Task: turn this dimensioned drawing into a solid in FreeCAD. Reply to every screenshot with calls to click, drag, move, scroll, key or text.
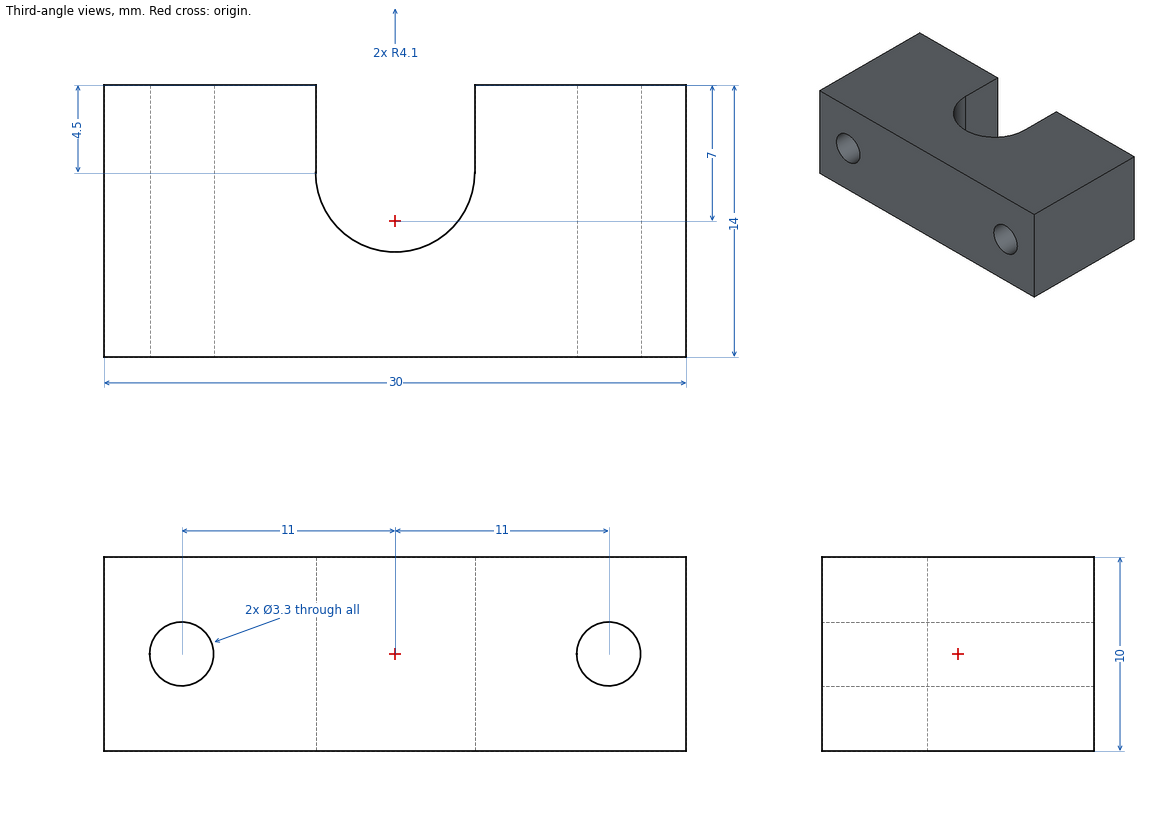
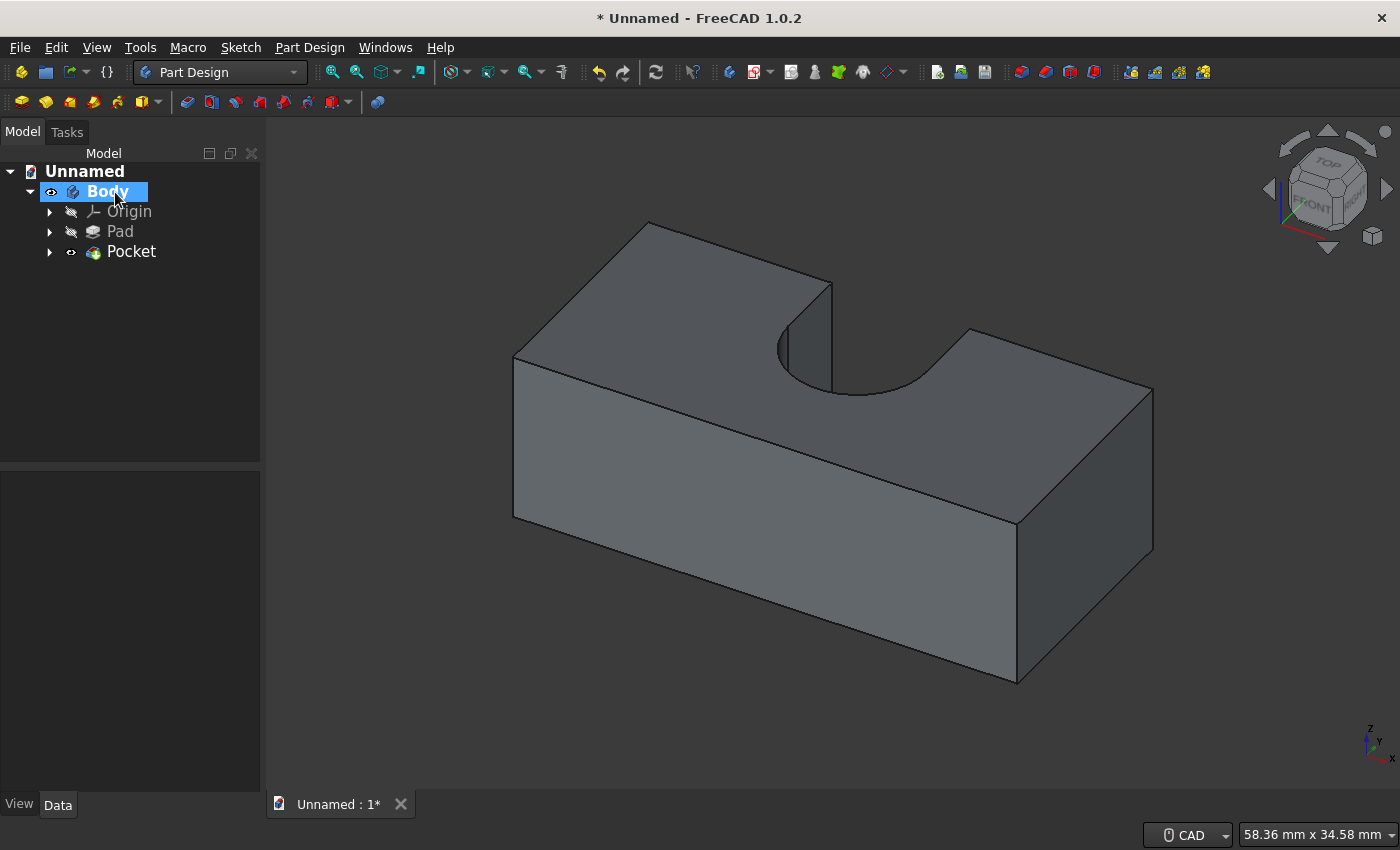
key(4)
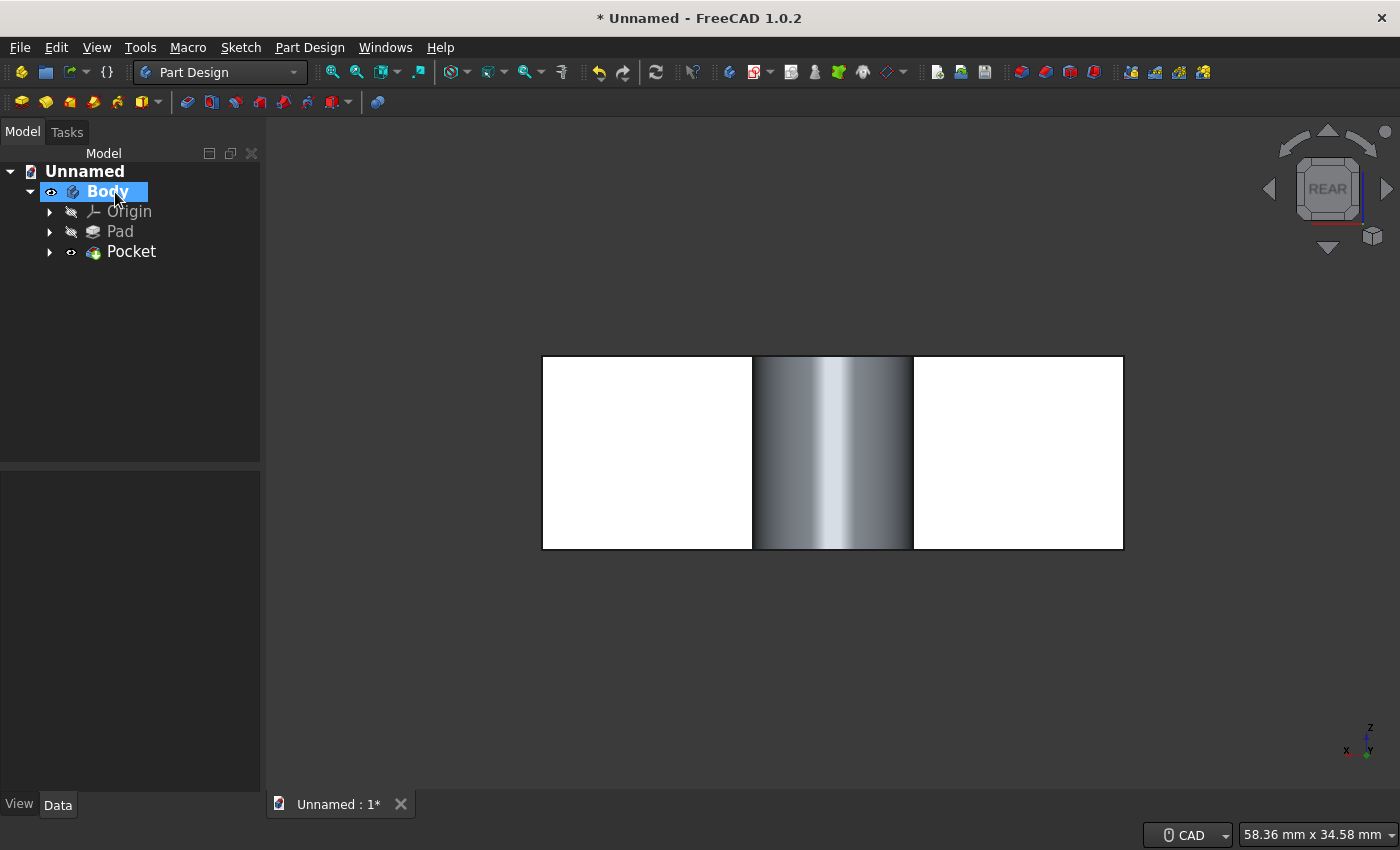
click(647, 452)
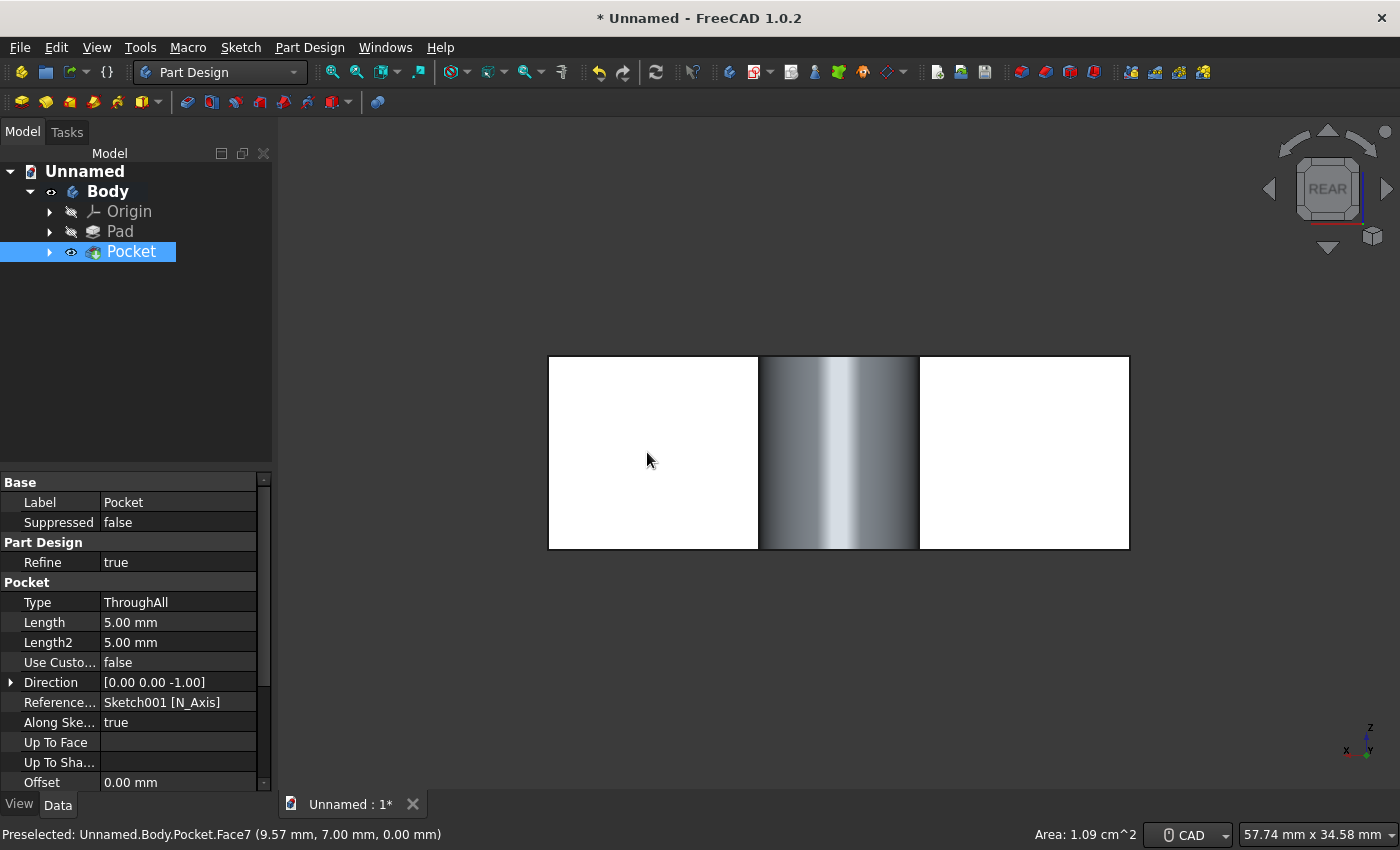
click(754, 72)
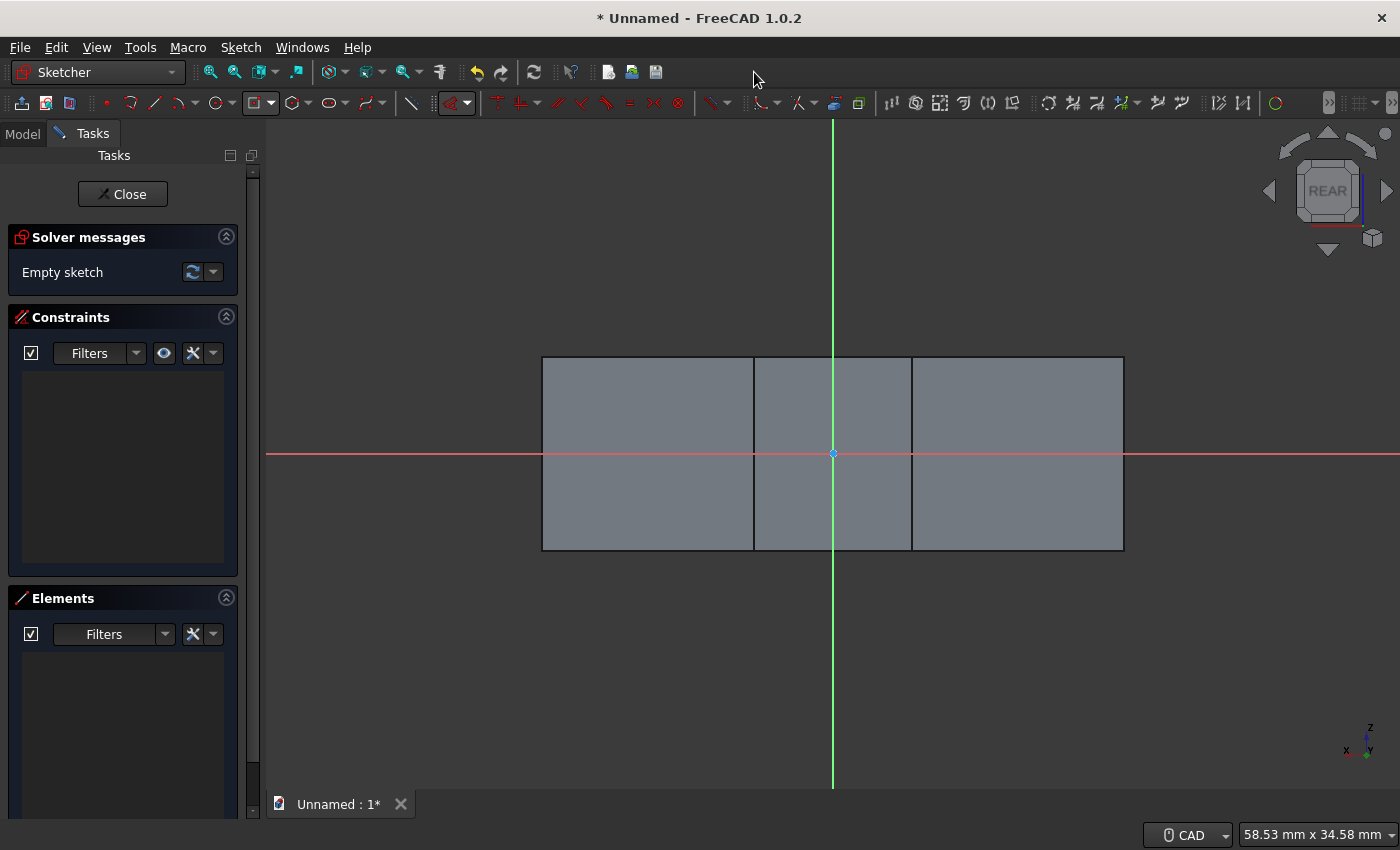
scroll(972, 454, up, 2)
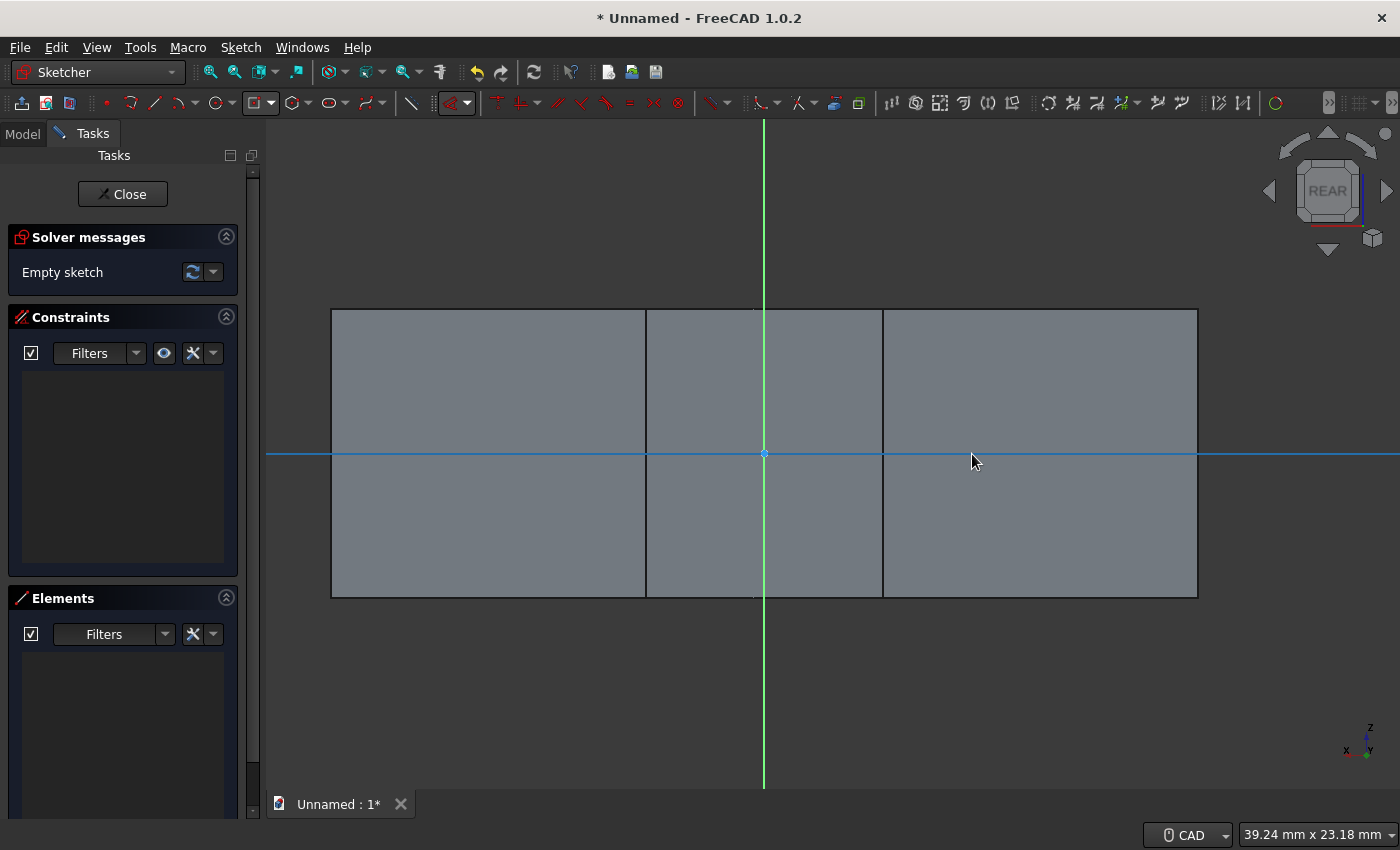
click(216, 104)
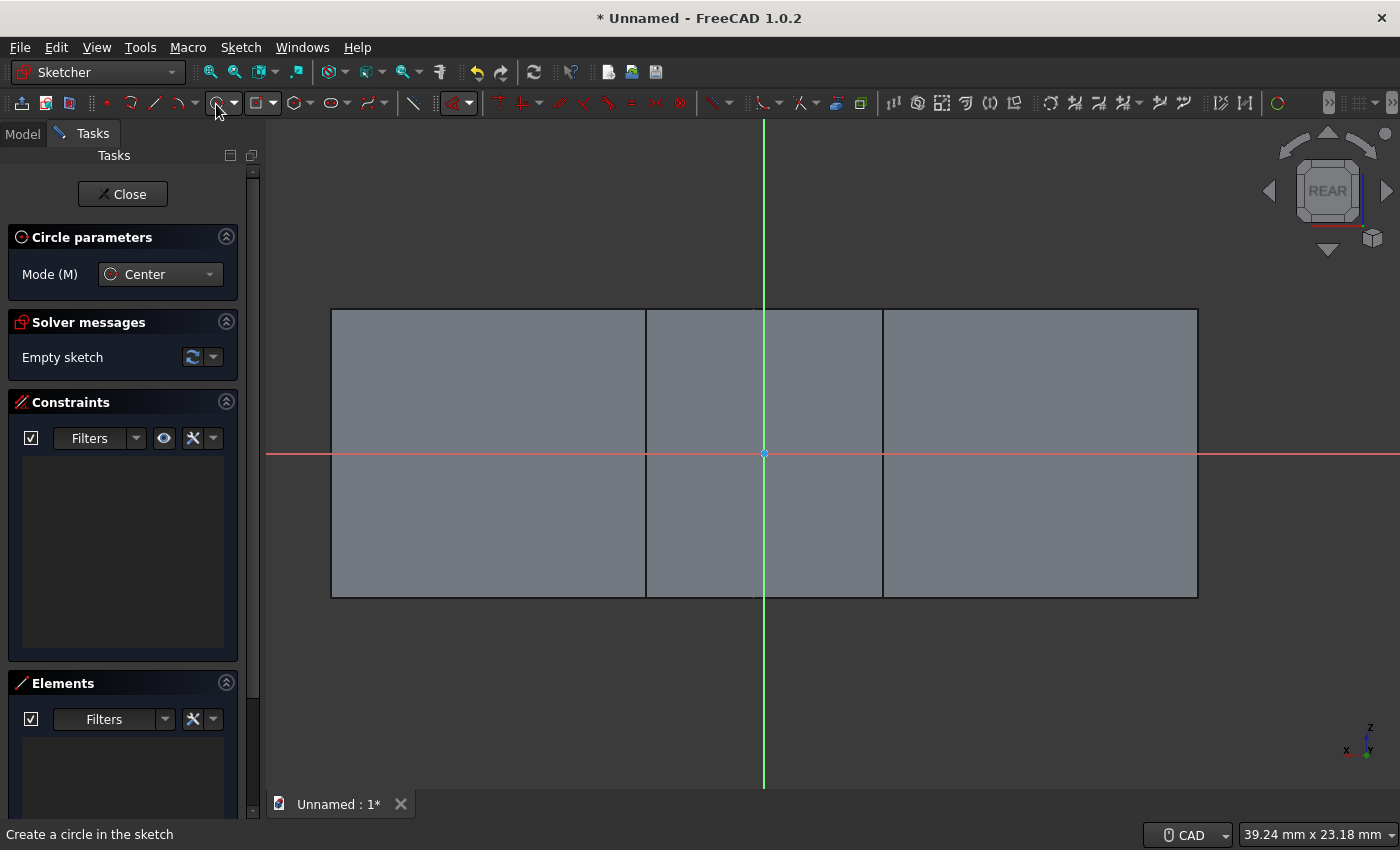
click(1082, 454)
move(1116, 420)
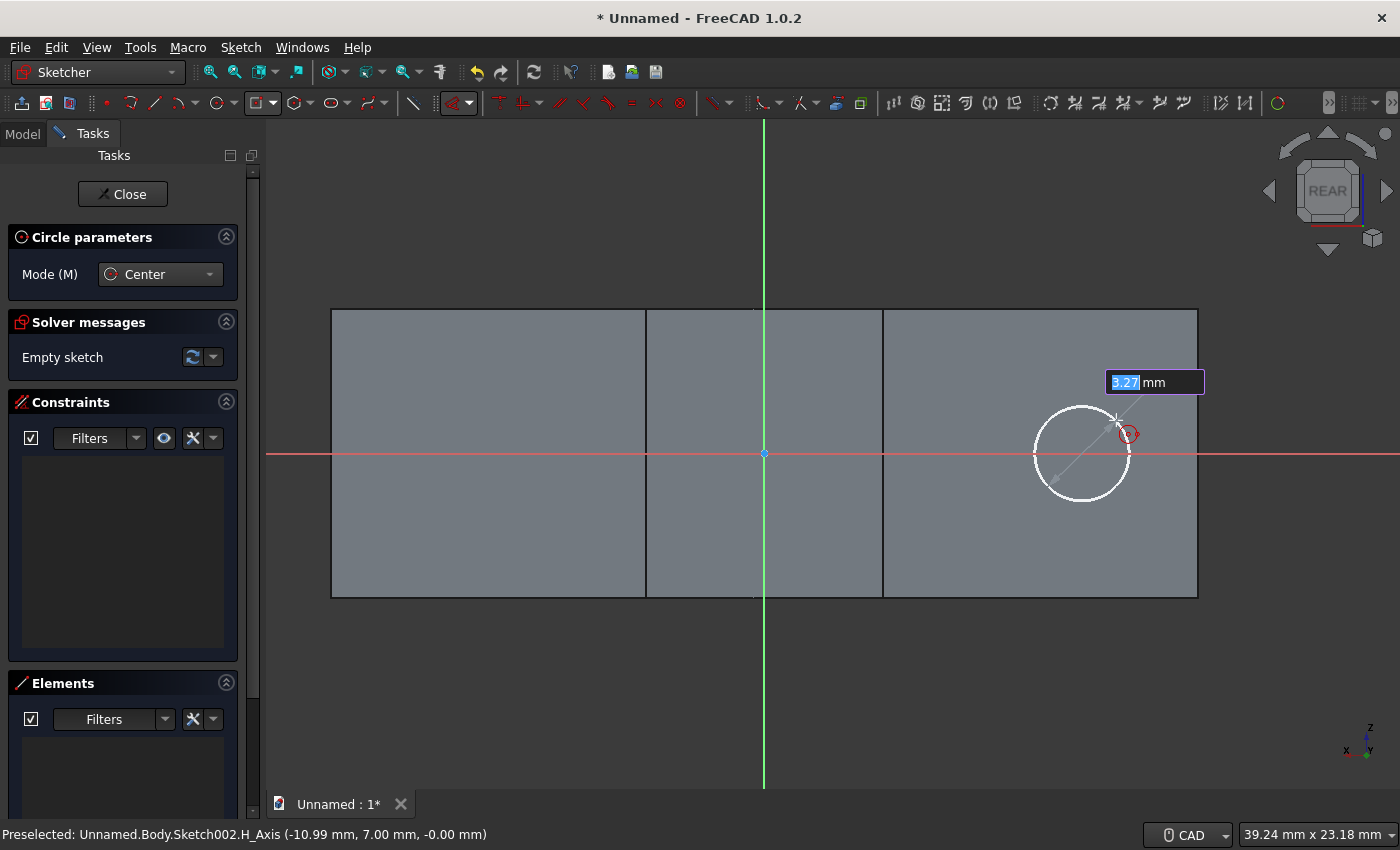
text(3.3)
key(Return)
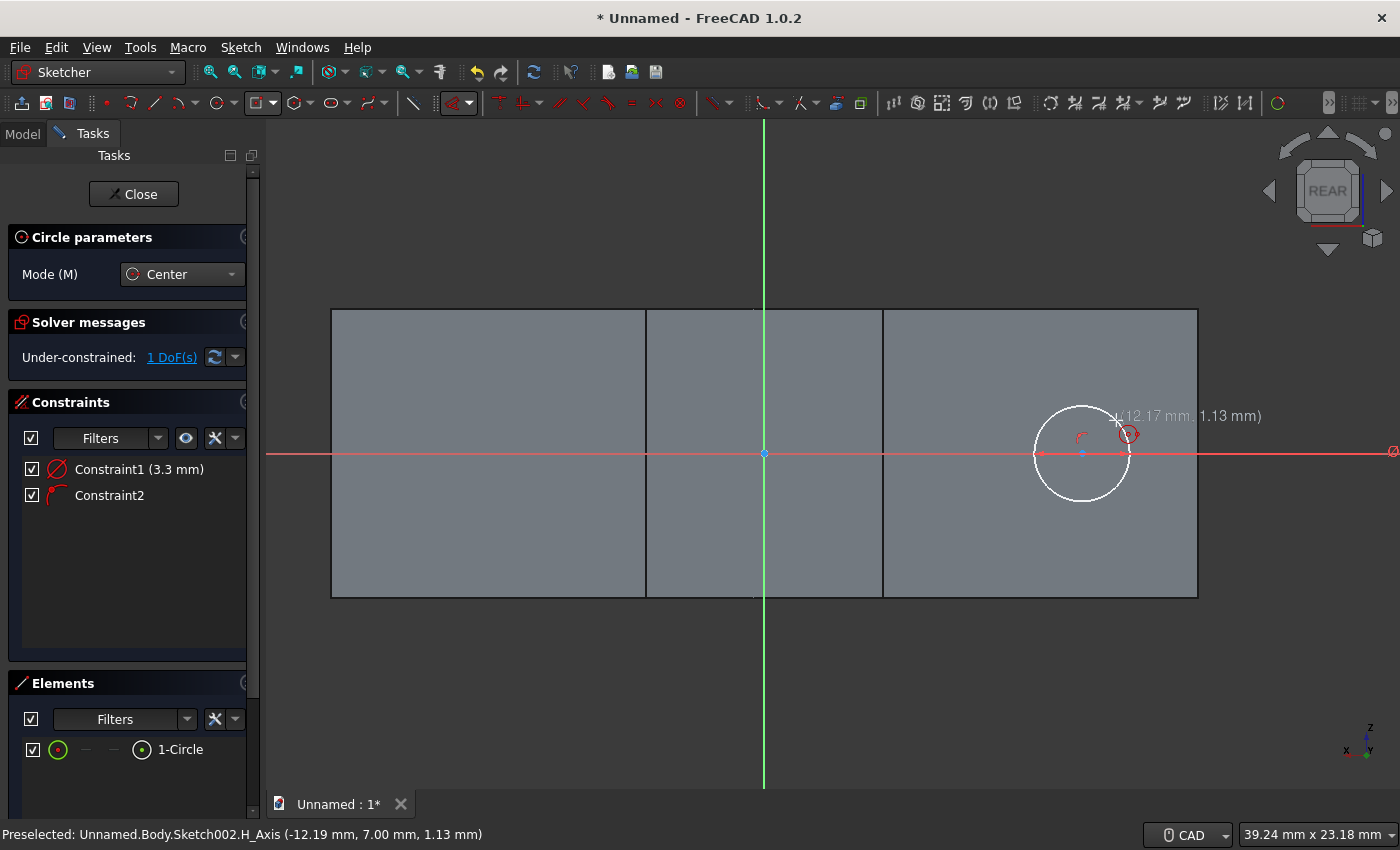
click(446, 454)
move(480, 420)